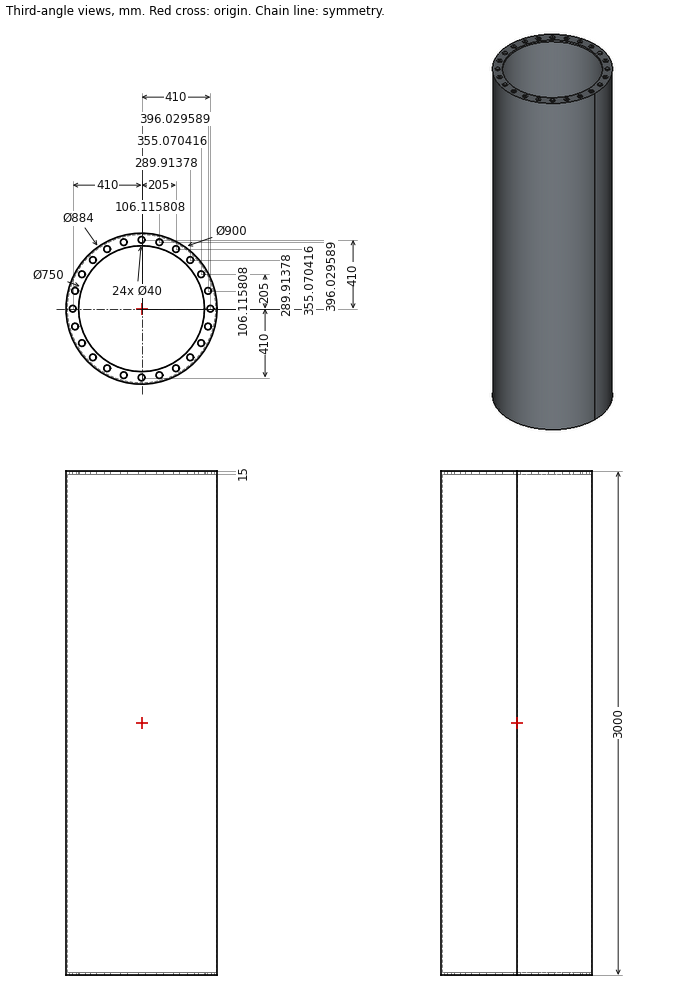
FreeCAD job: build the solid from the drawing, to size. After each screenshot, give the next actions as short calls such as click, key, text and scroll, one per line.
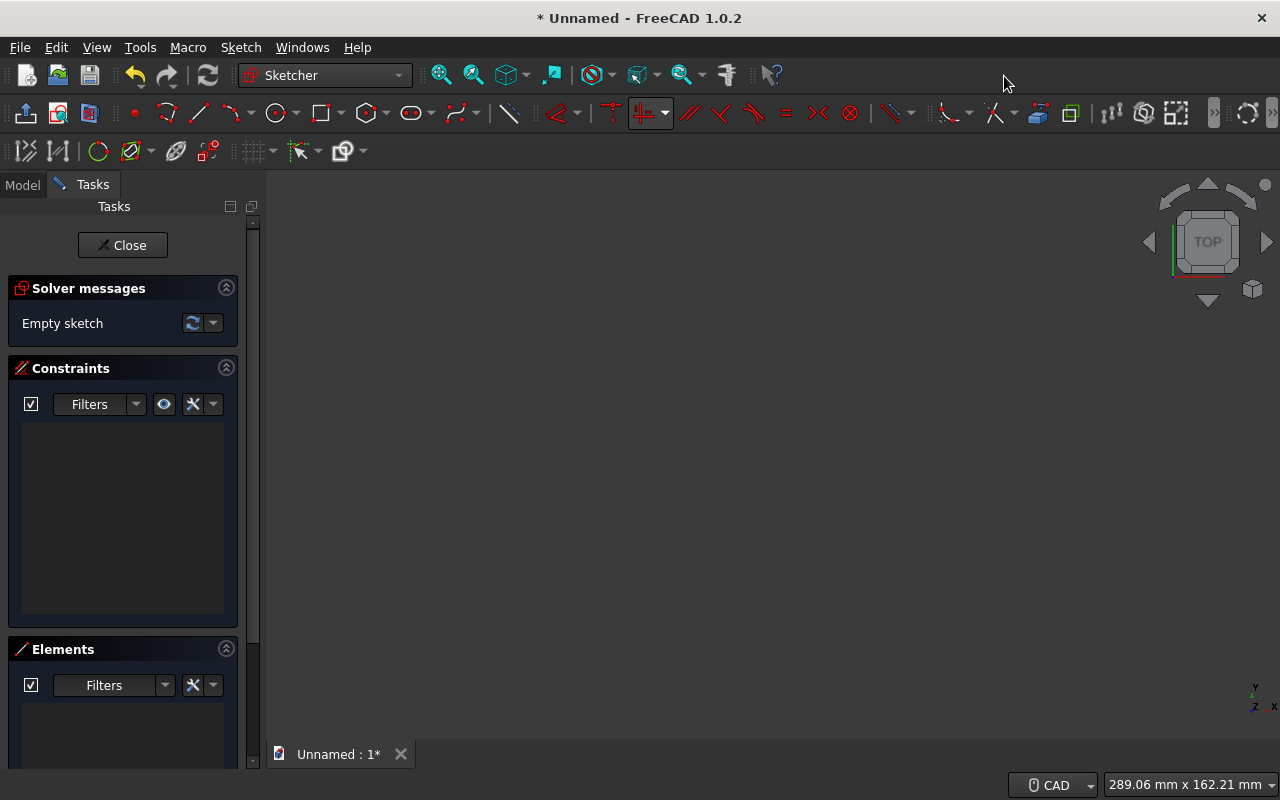
scroll(629, 198, down, 12)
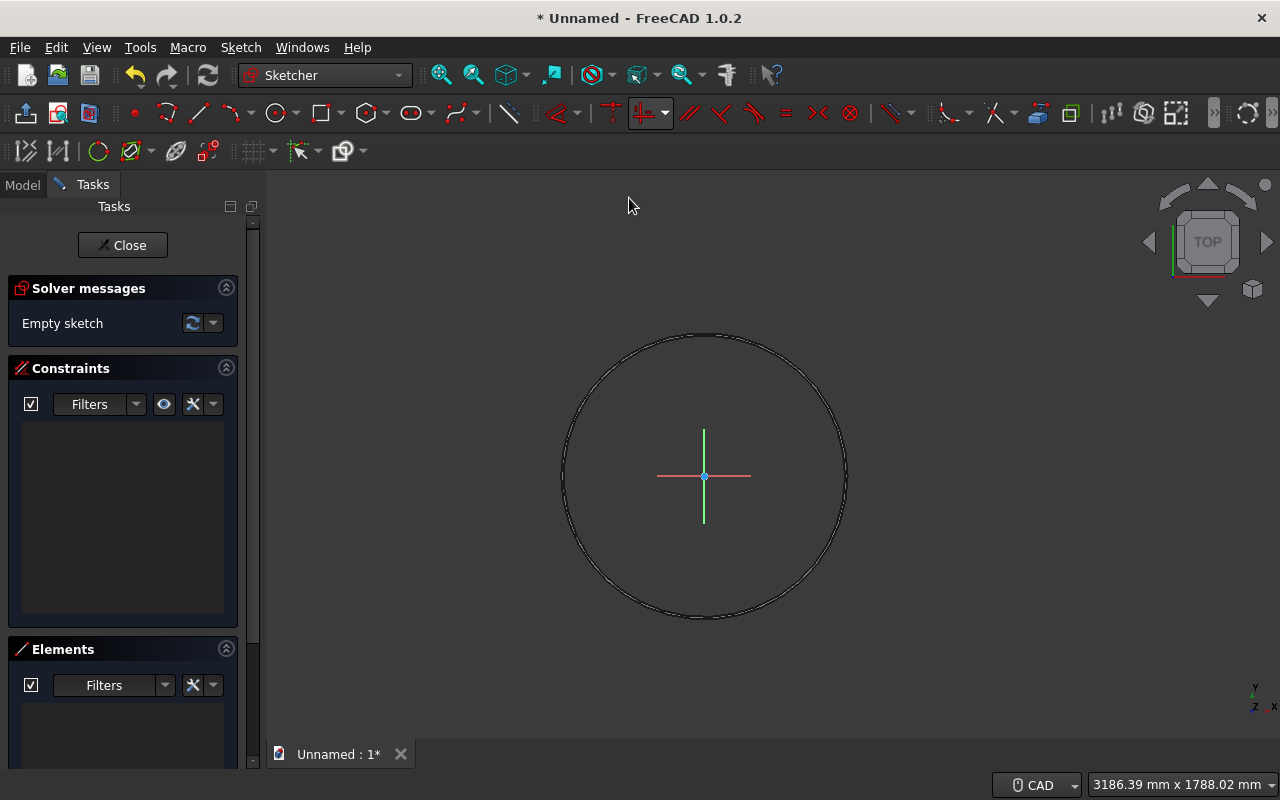
click(276, 114)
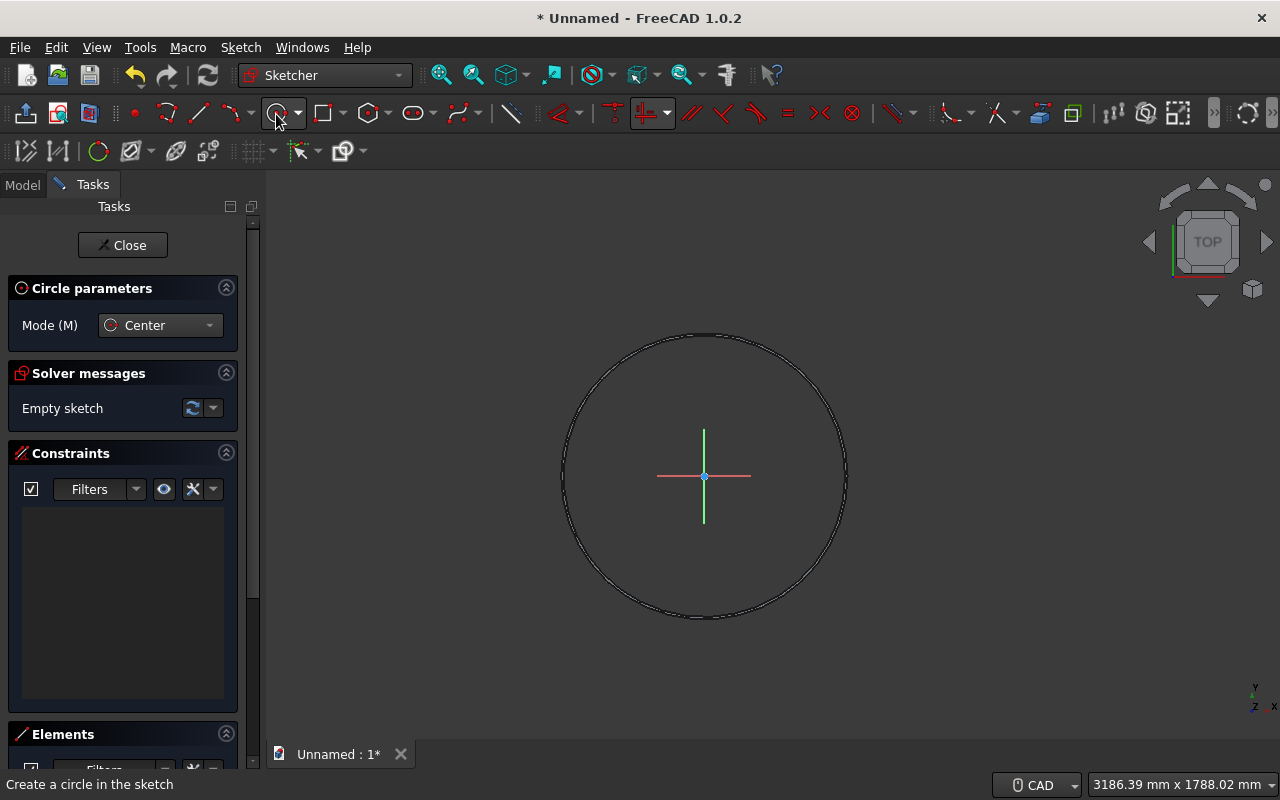
click(704, 476)
move(806, 375)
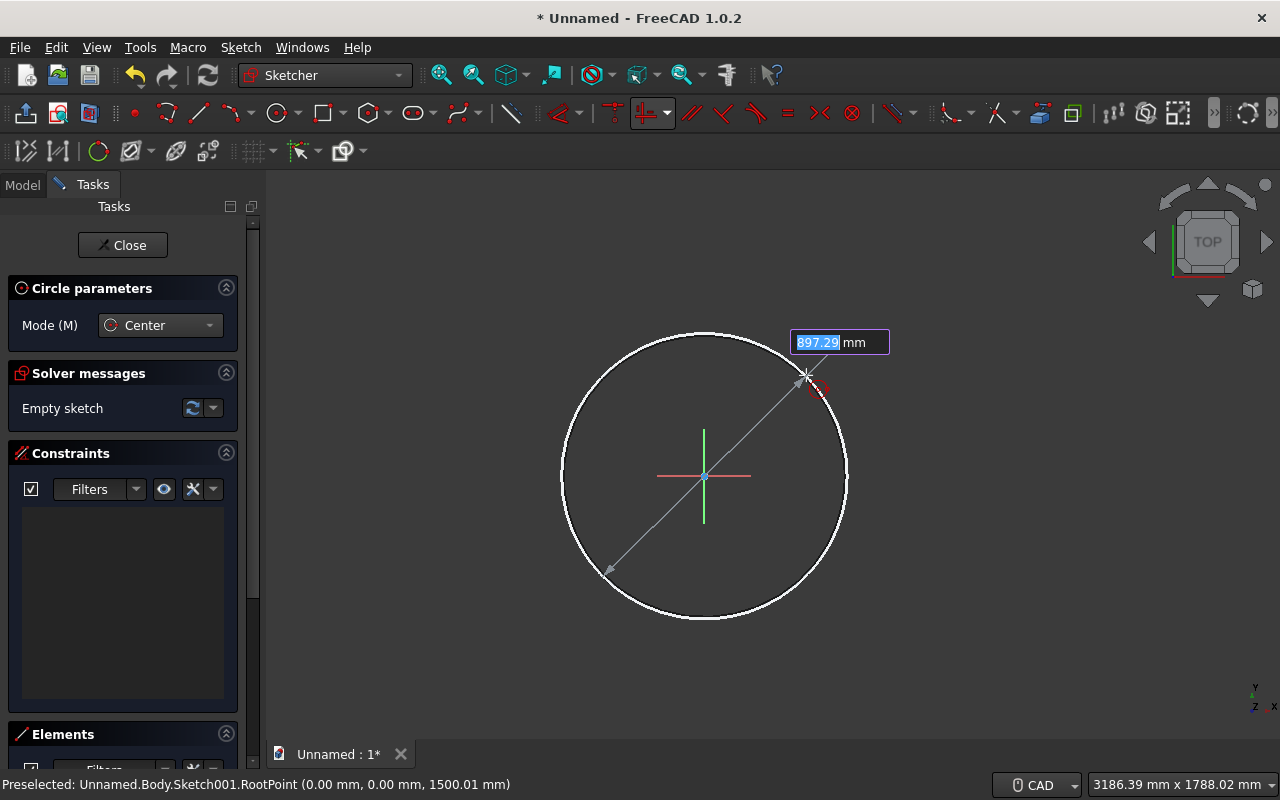
text(900)
key(Return)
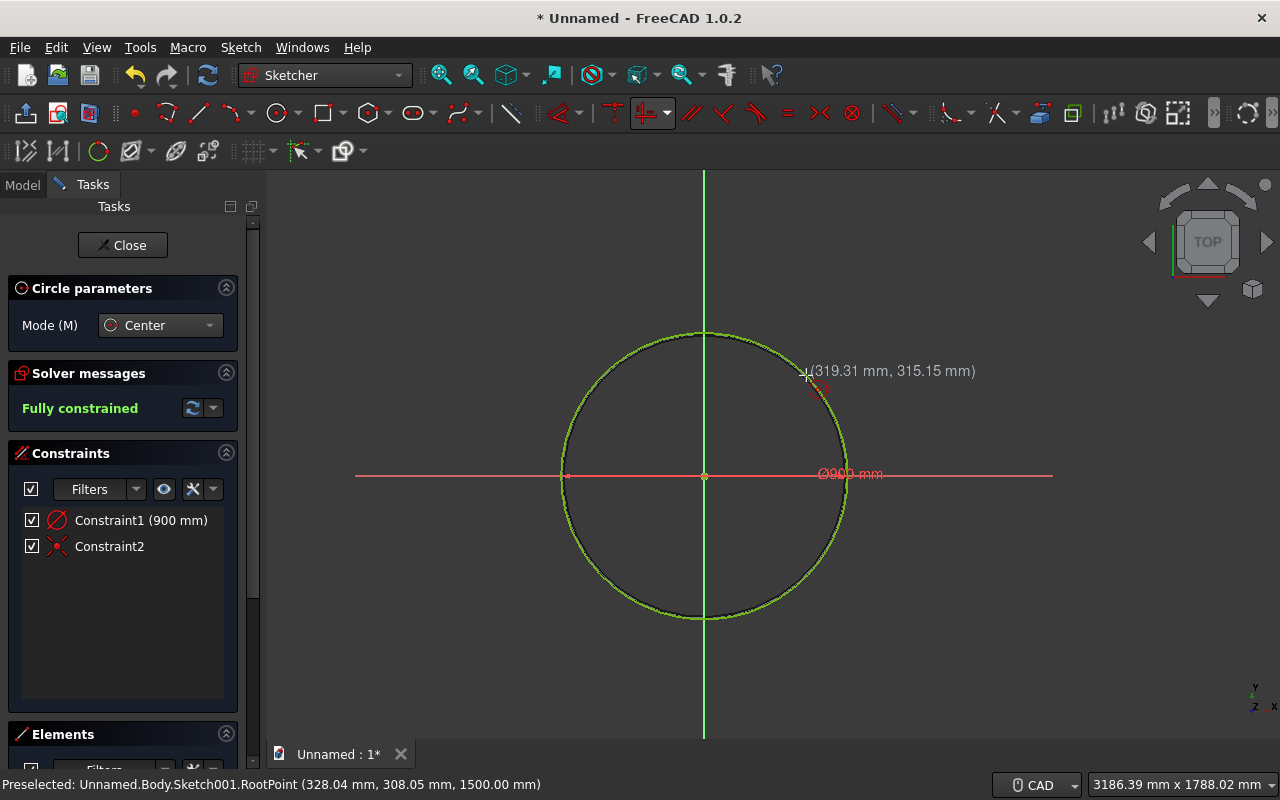
click(704, 476)
move(789, 392)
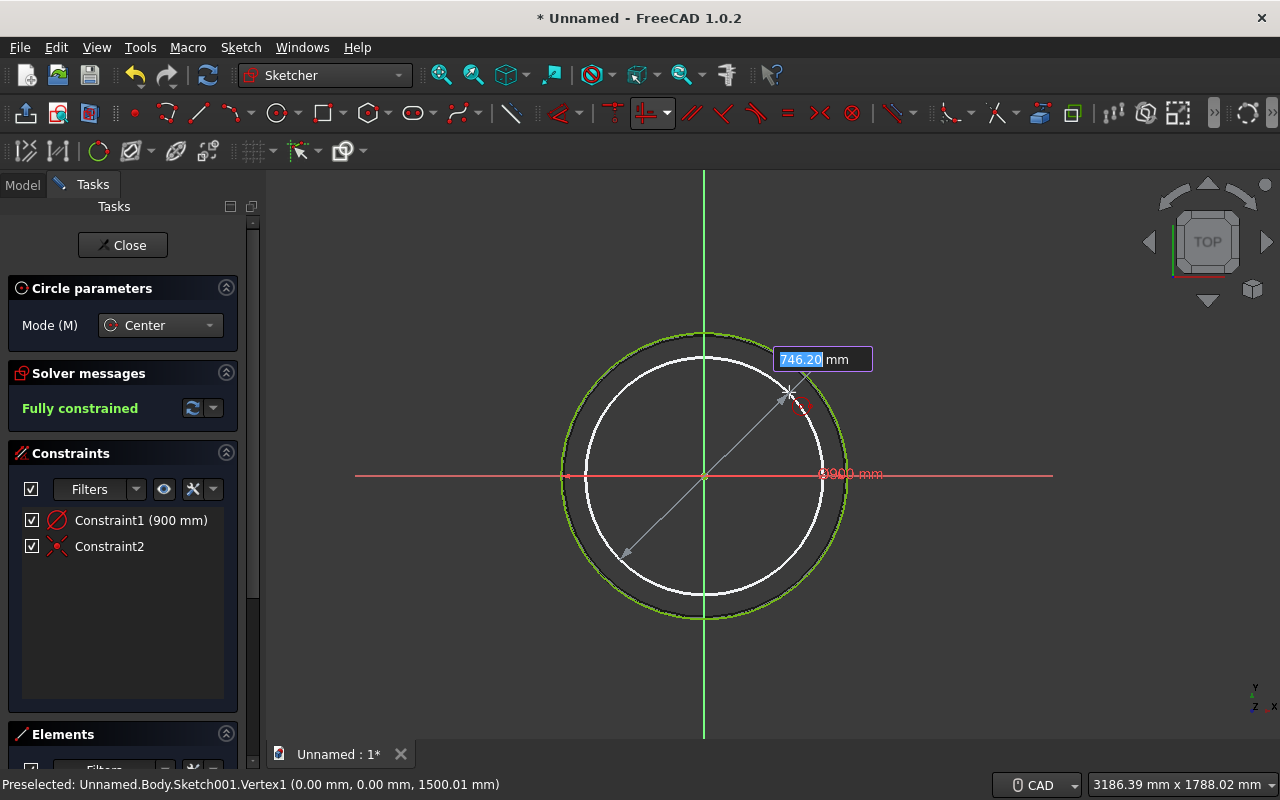
text(750)
key(Return)
key(Escape)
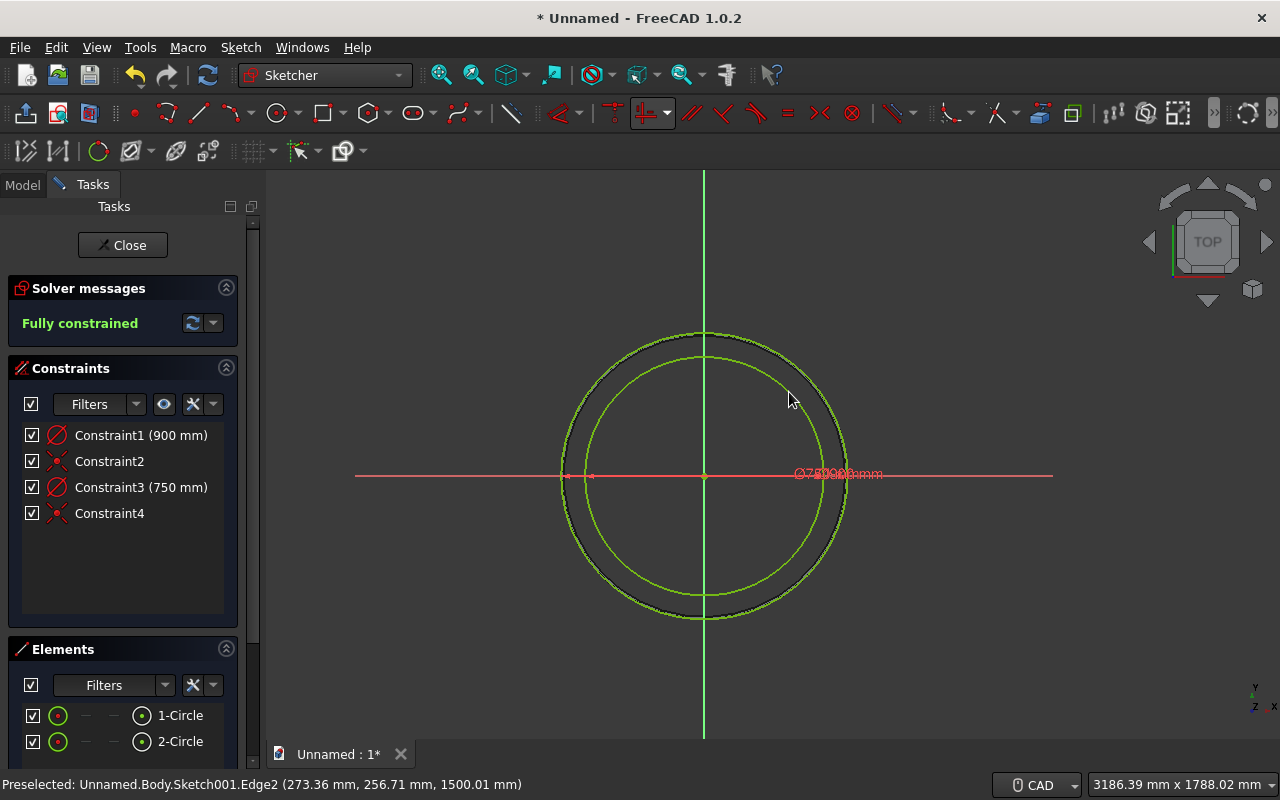
click(123, 245)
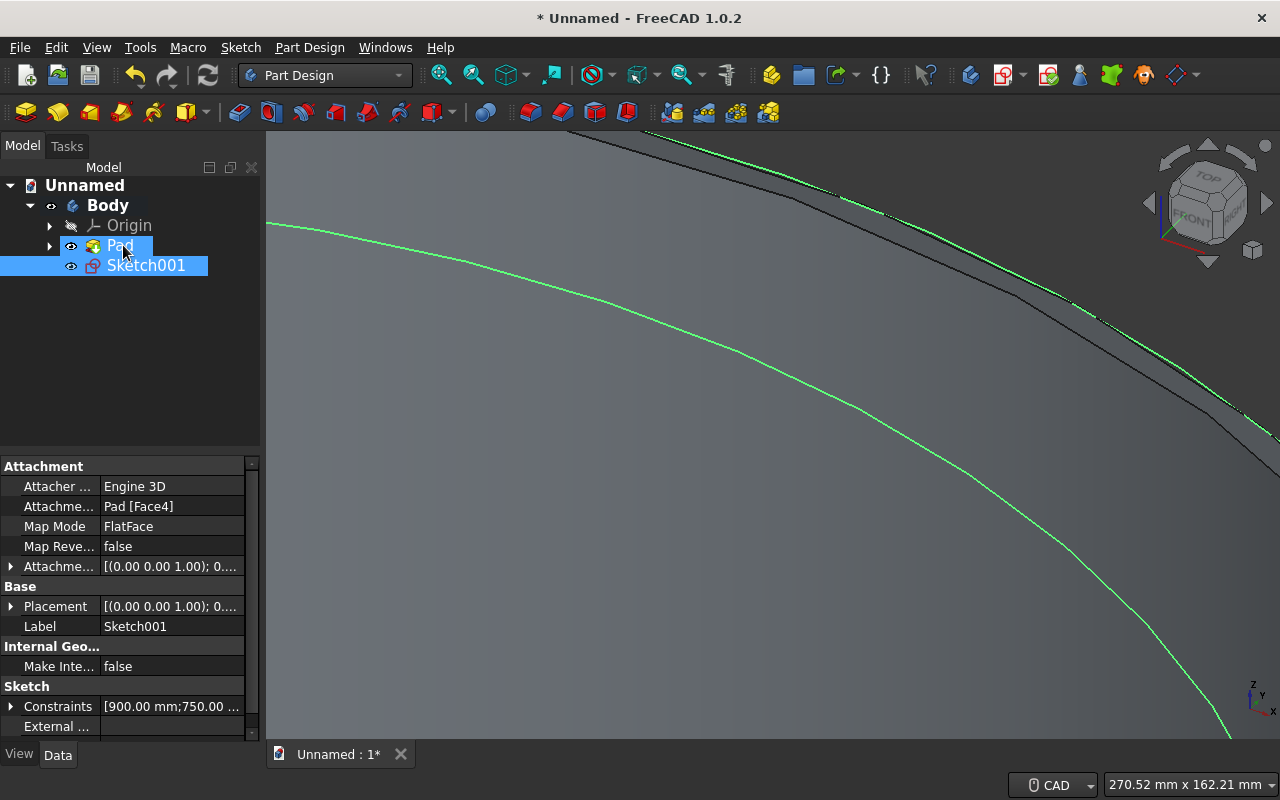
click(26, 112)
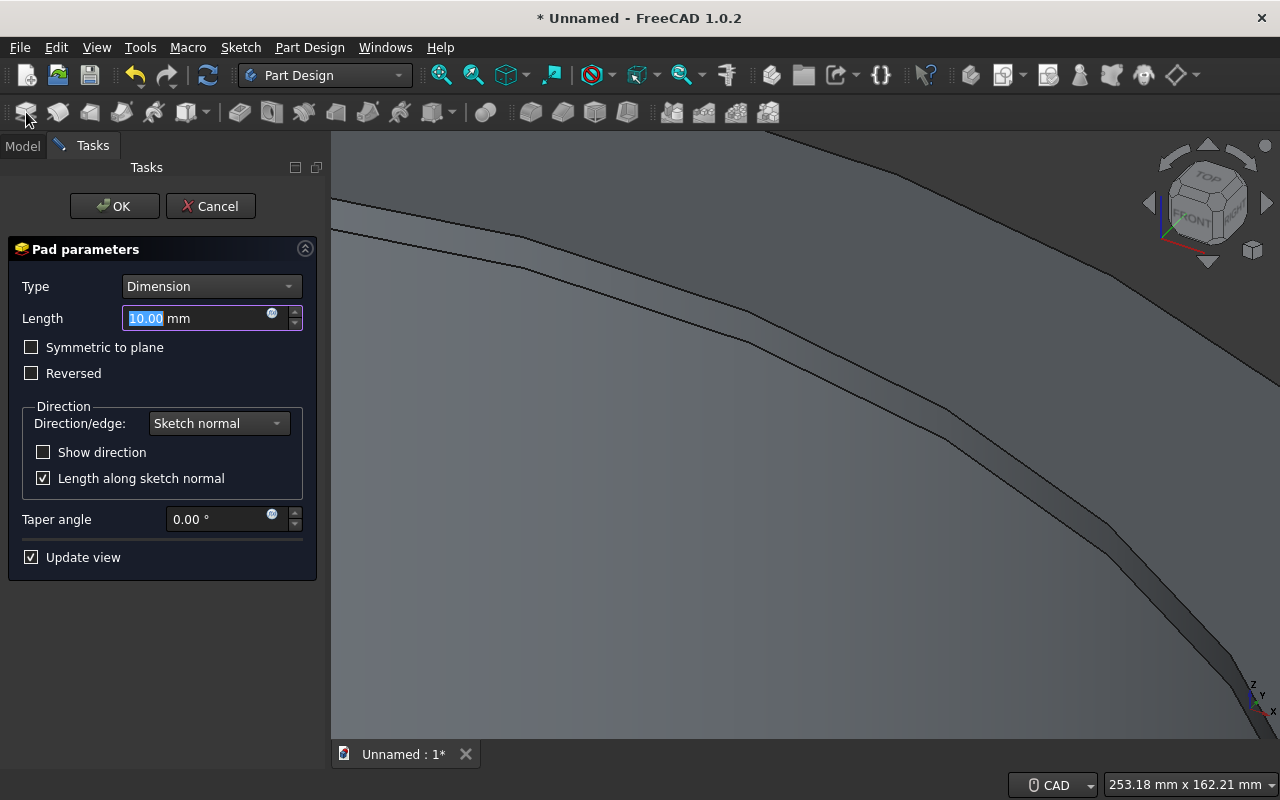
text(15)
key(Tab)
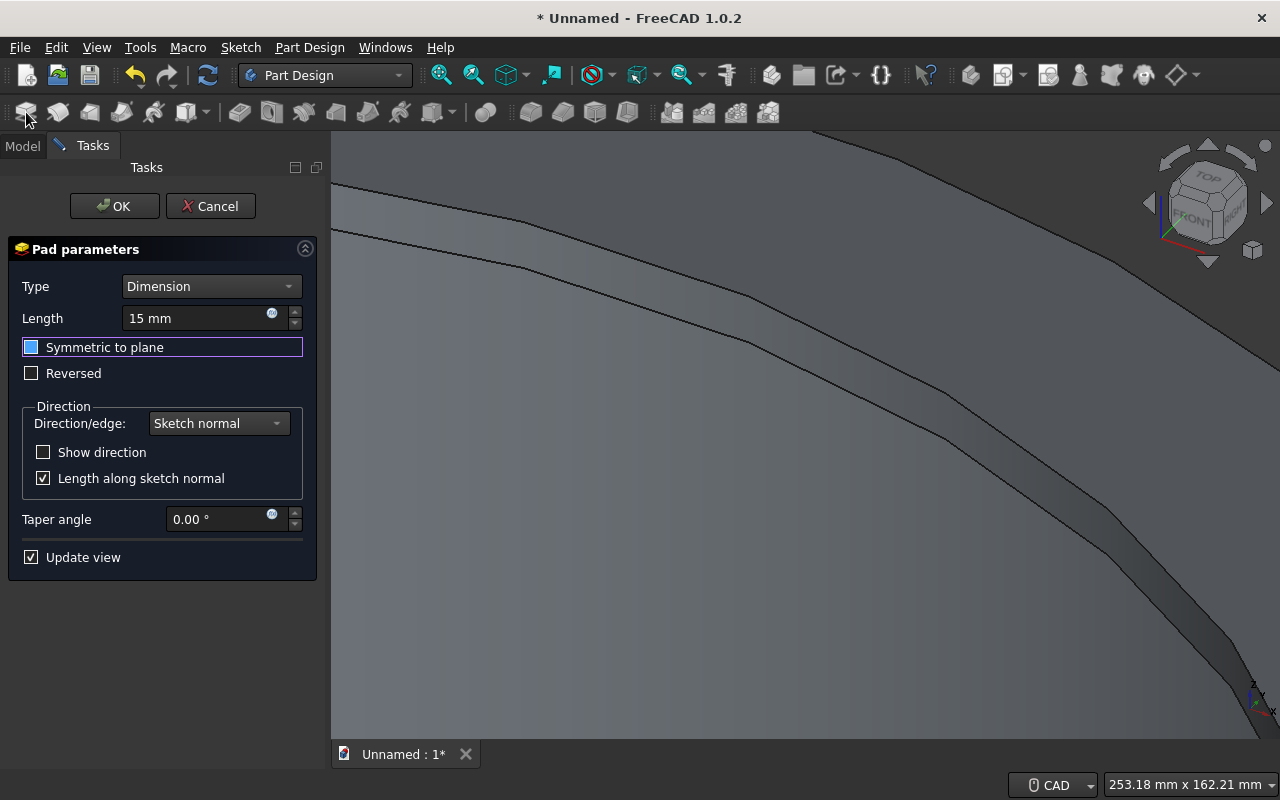
click(30, 373)